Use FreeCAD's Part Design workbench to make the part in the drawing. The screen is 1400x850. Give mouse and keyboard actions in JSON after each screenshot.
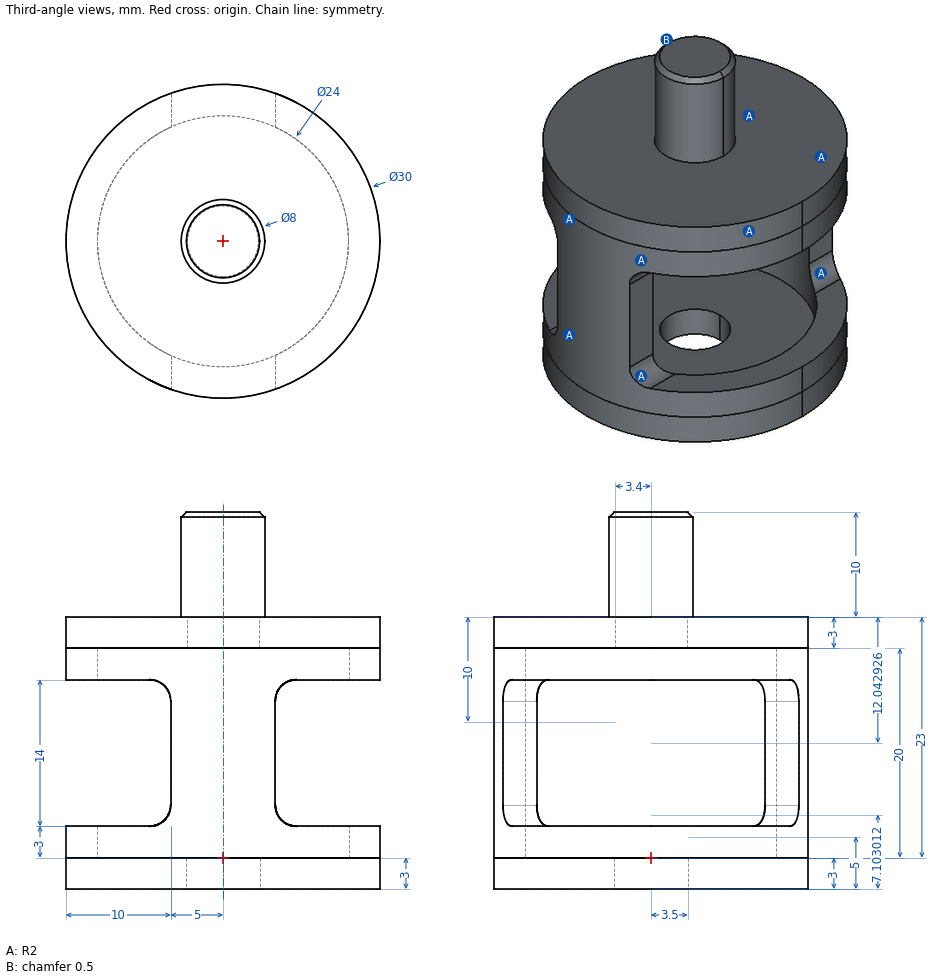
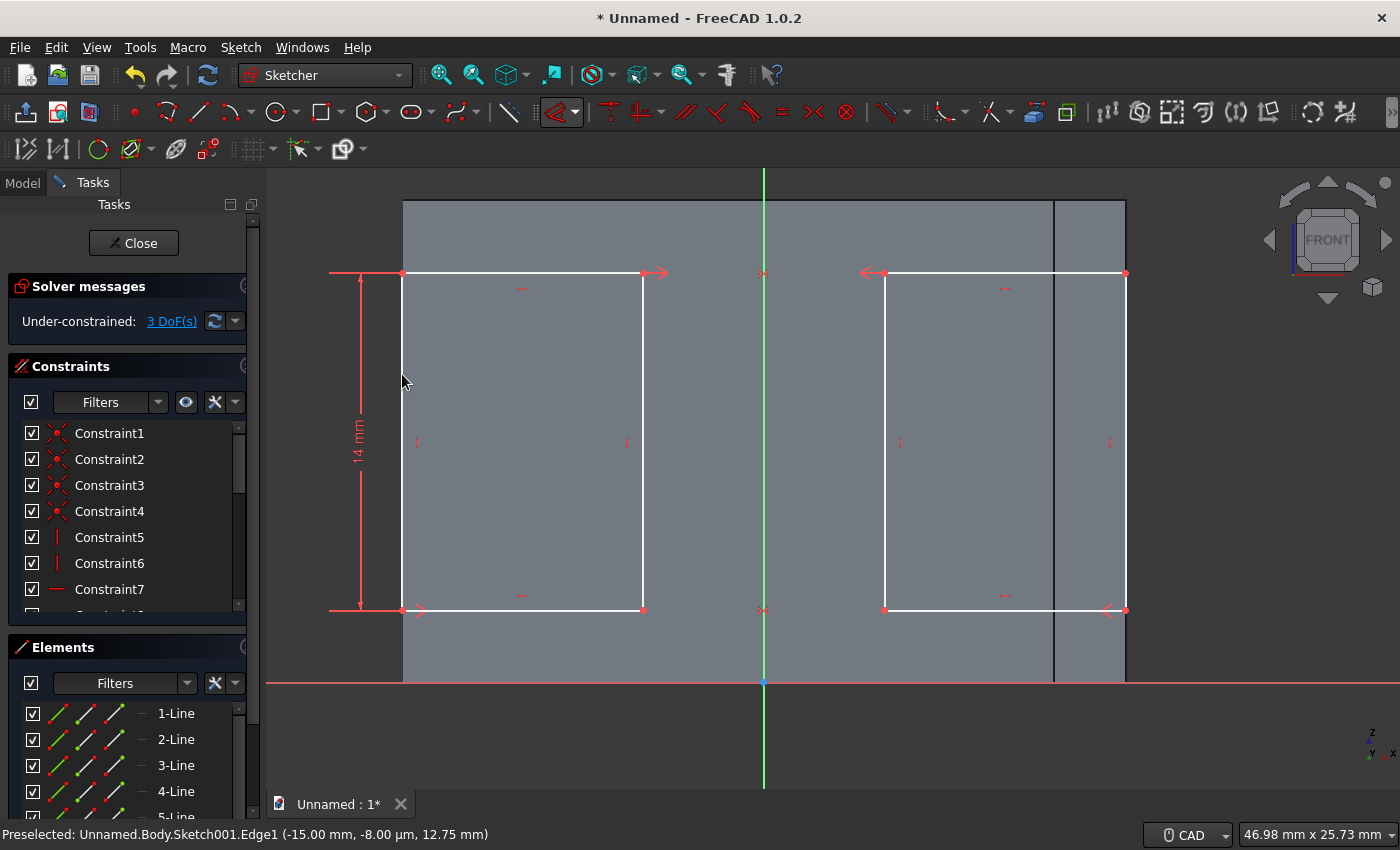
{"action": "left_click", "coordinate": [474, 611]}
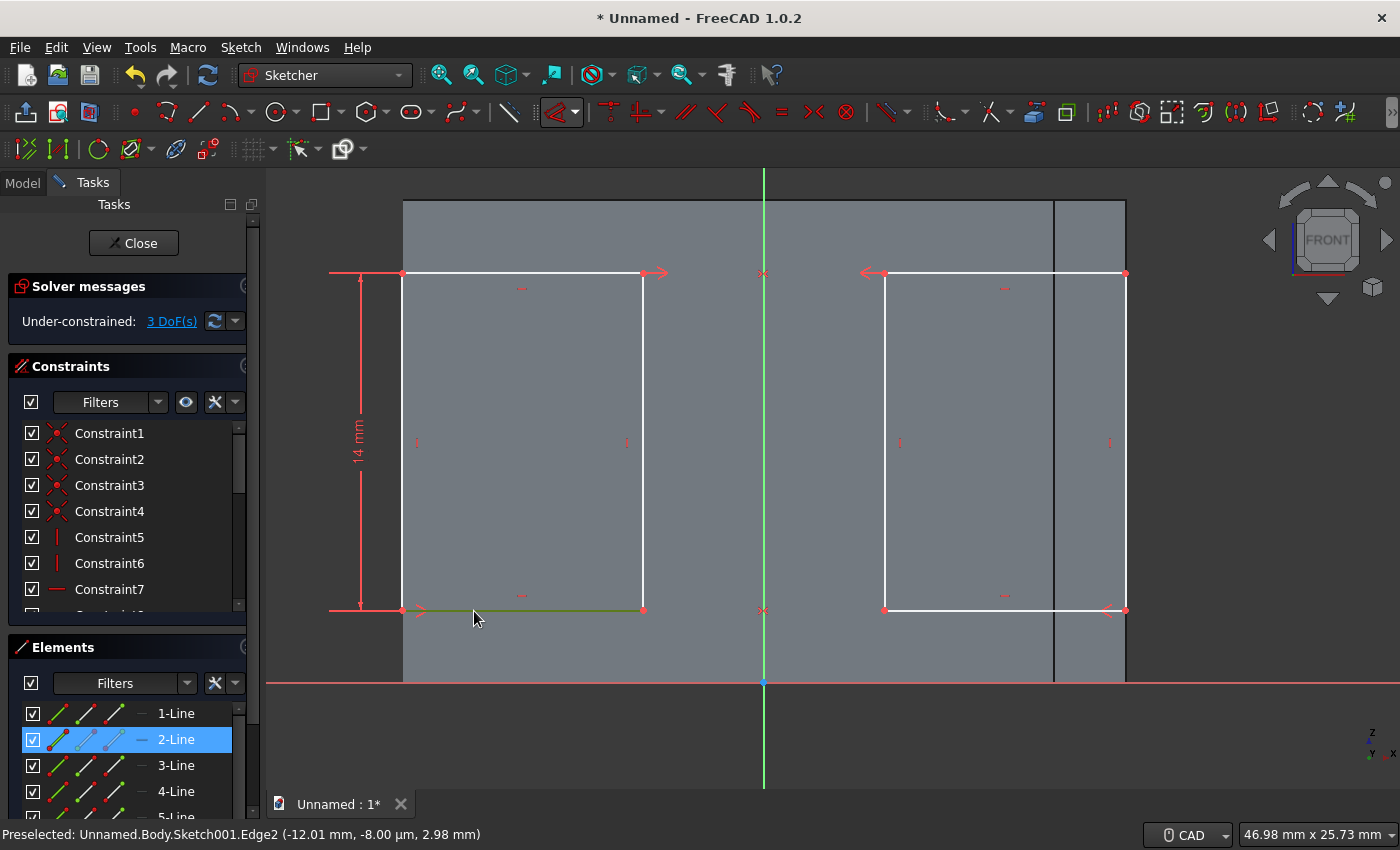
{"action": "key", "text": "l"}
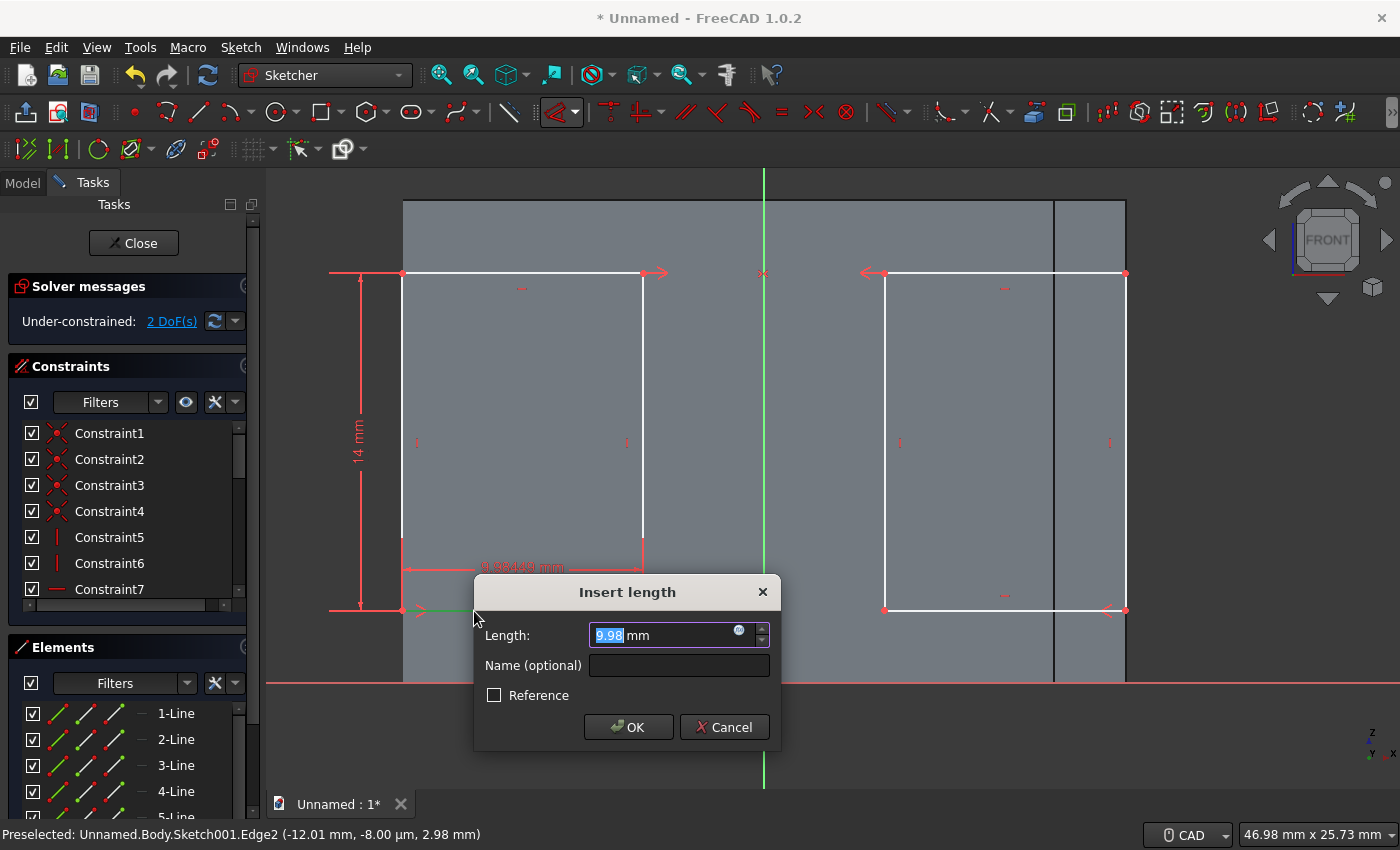
{"action": "type", "text": "10"}
{"action": "key", "text": "Return"}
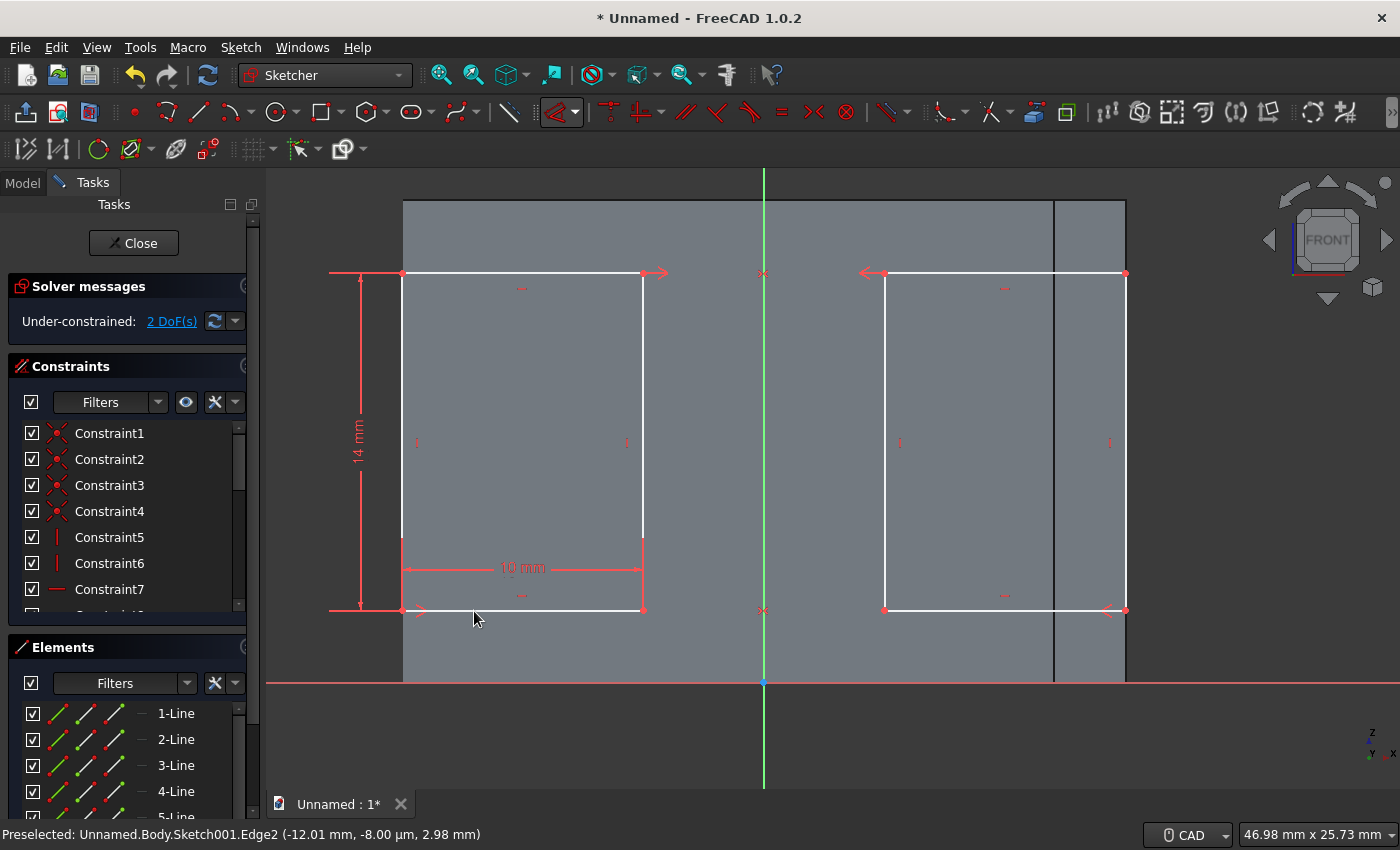
{"action": "left_click", "coordinate": [402, 611]}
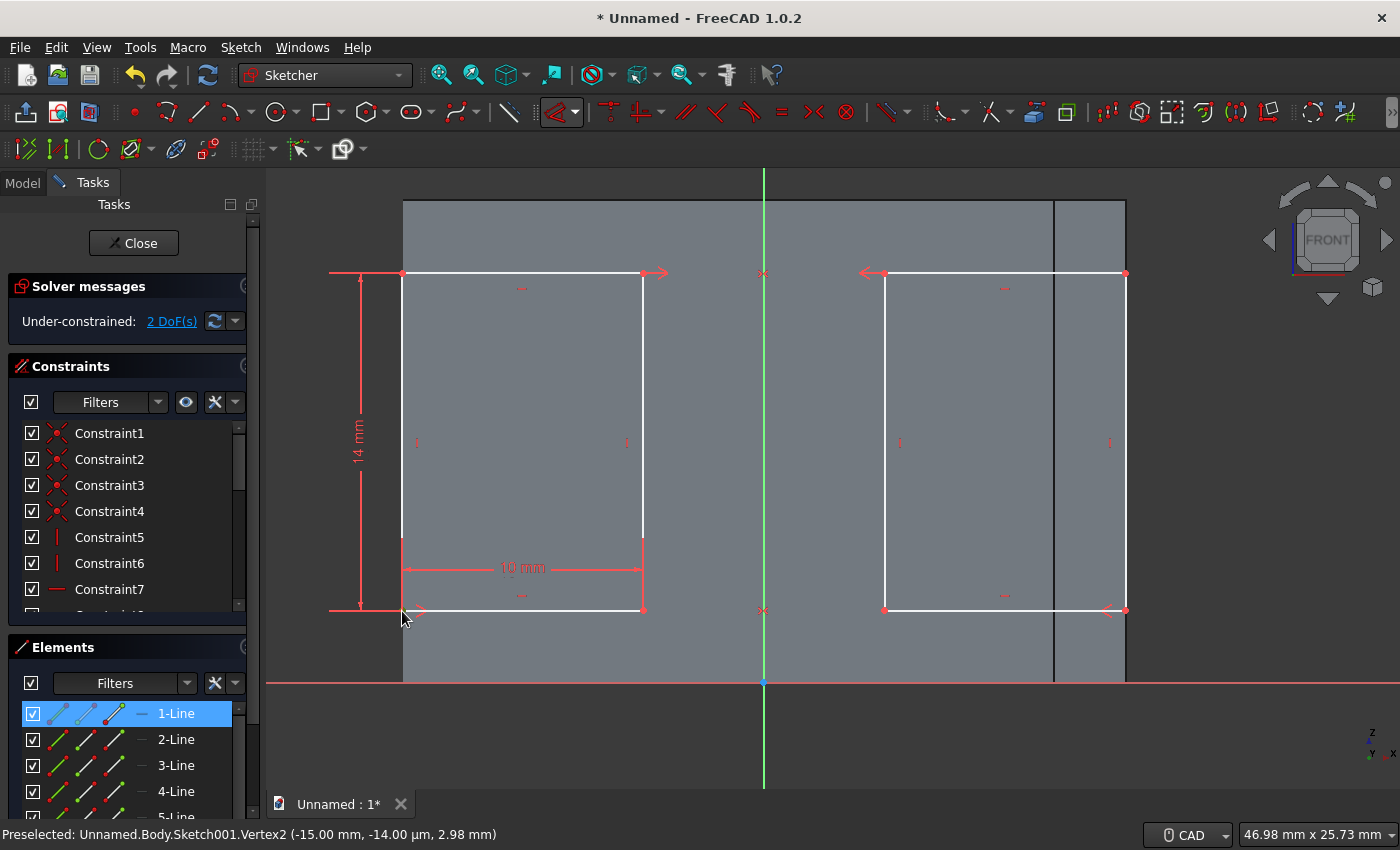
{"action": "key", "text": "i"}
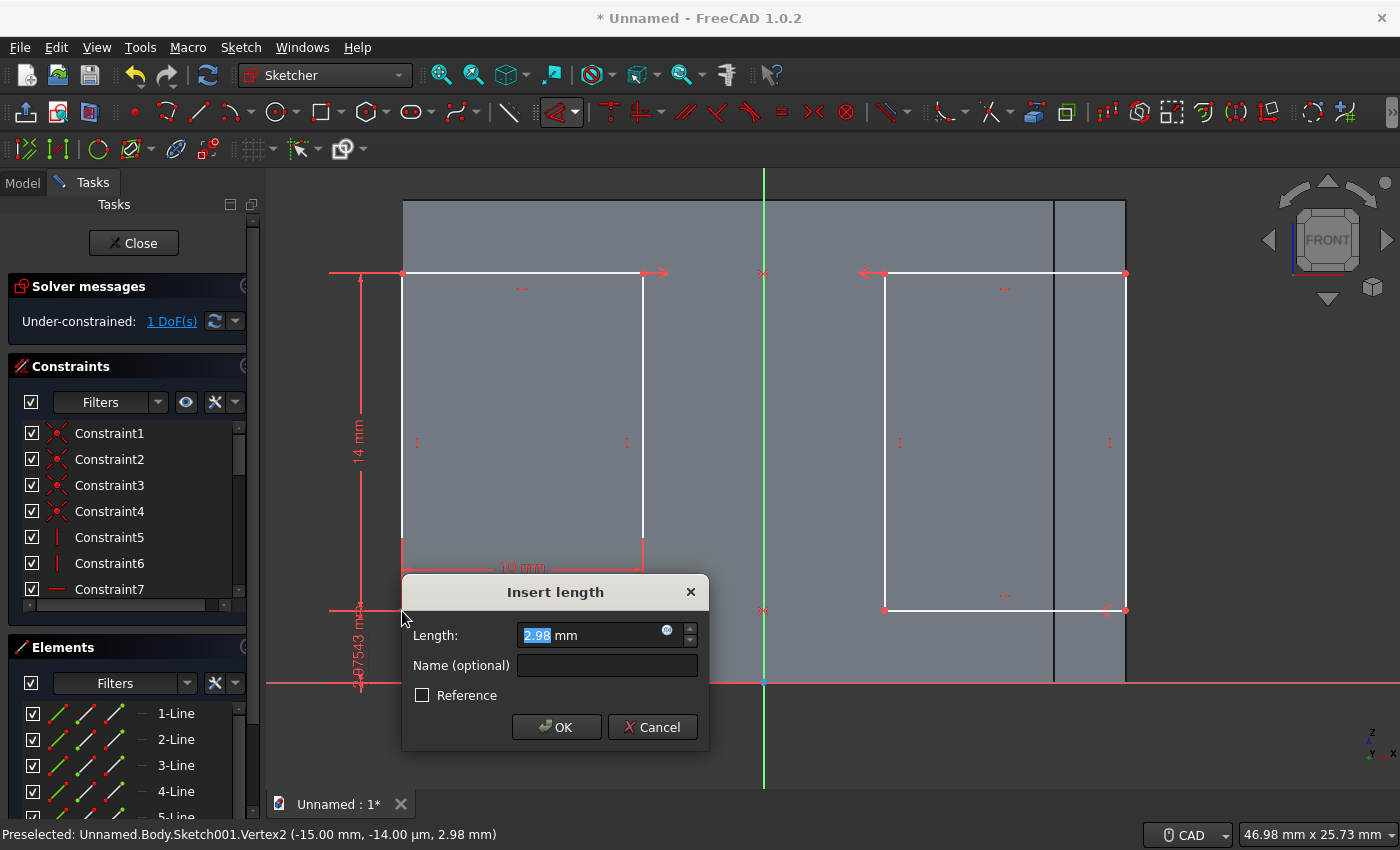
{"action": "type", "text": "3"}
{"action": "key", "text": "Return"}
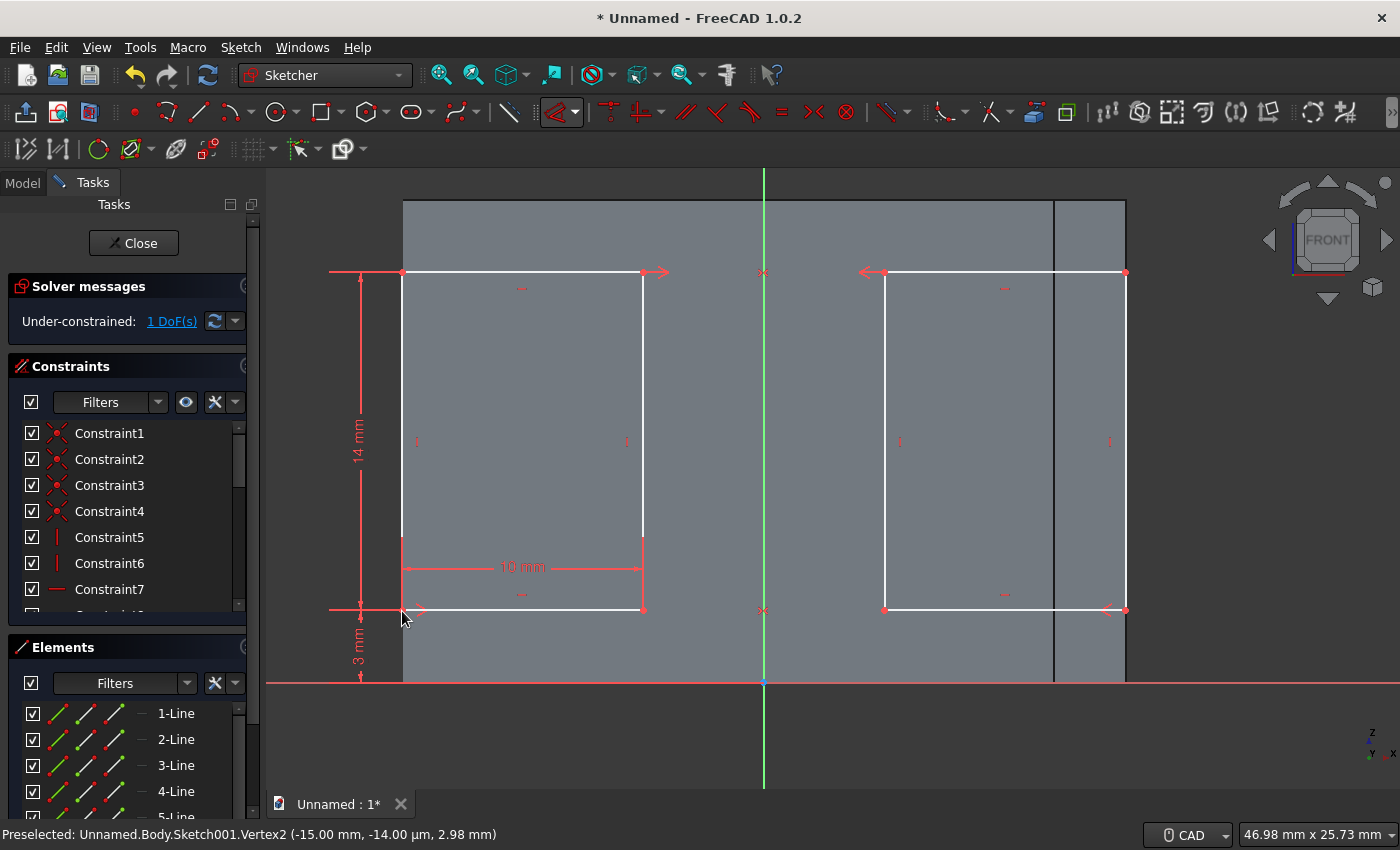
{"action": "left_click", "coordinate": [643, 610]}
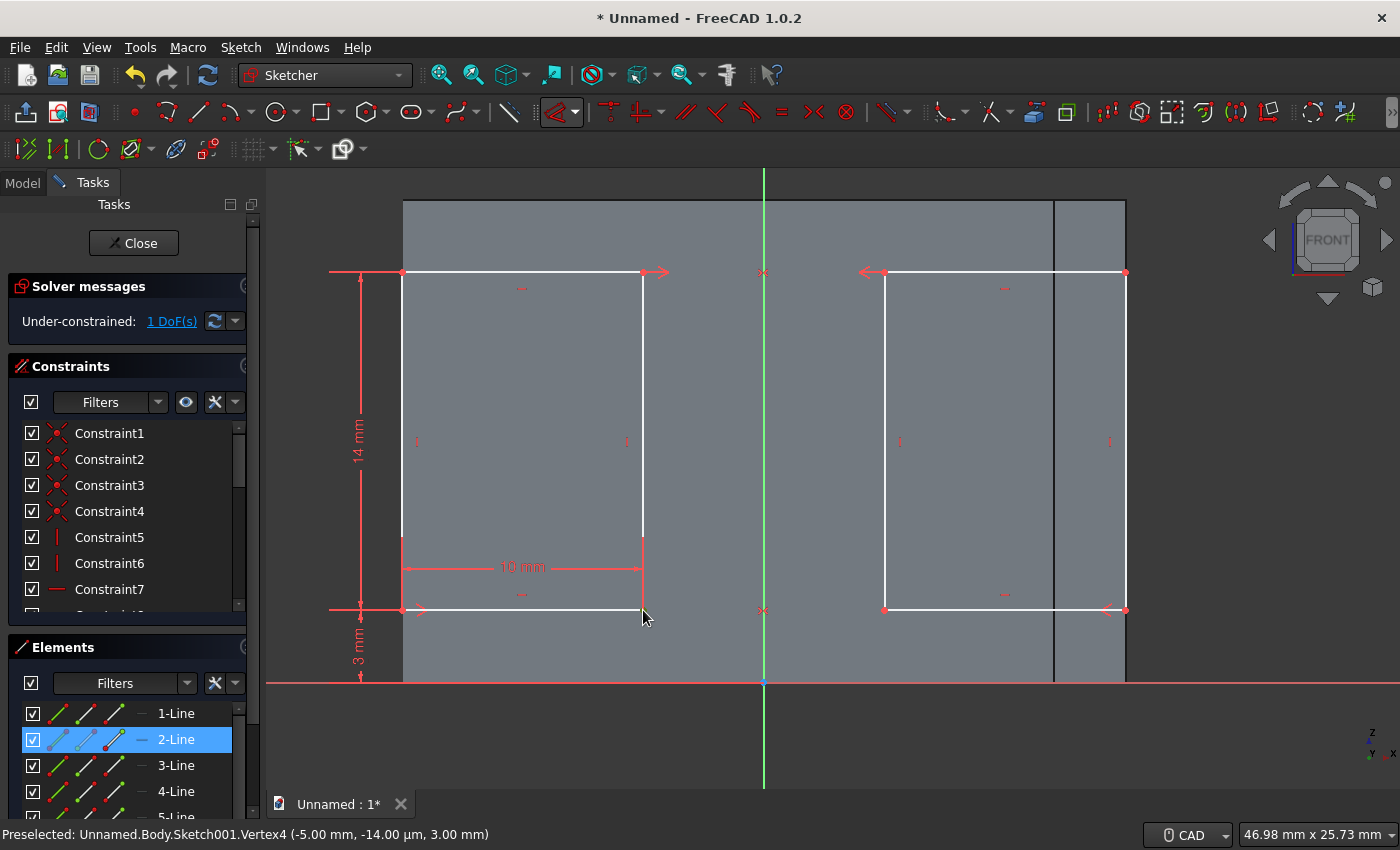
{"action": "key", "text": "l"}